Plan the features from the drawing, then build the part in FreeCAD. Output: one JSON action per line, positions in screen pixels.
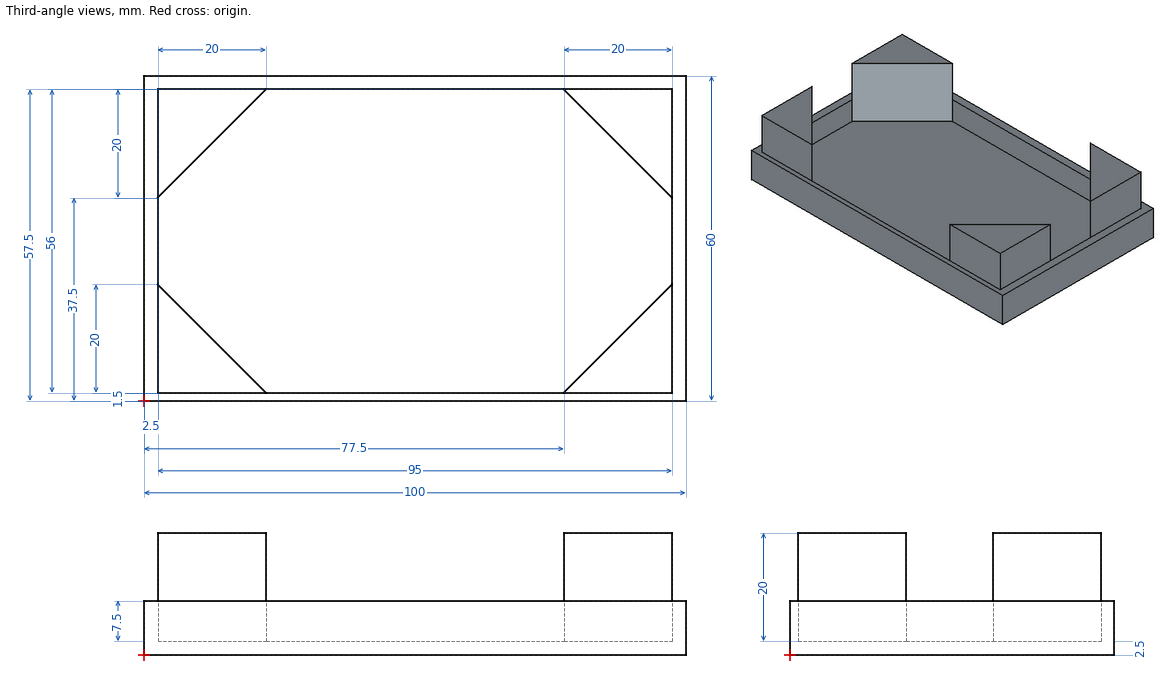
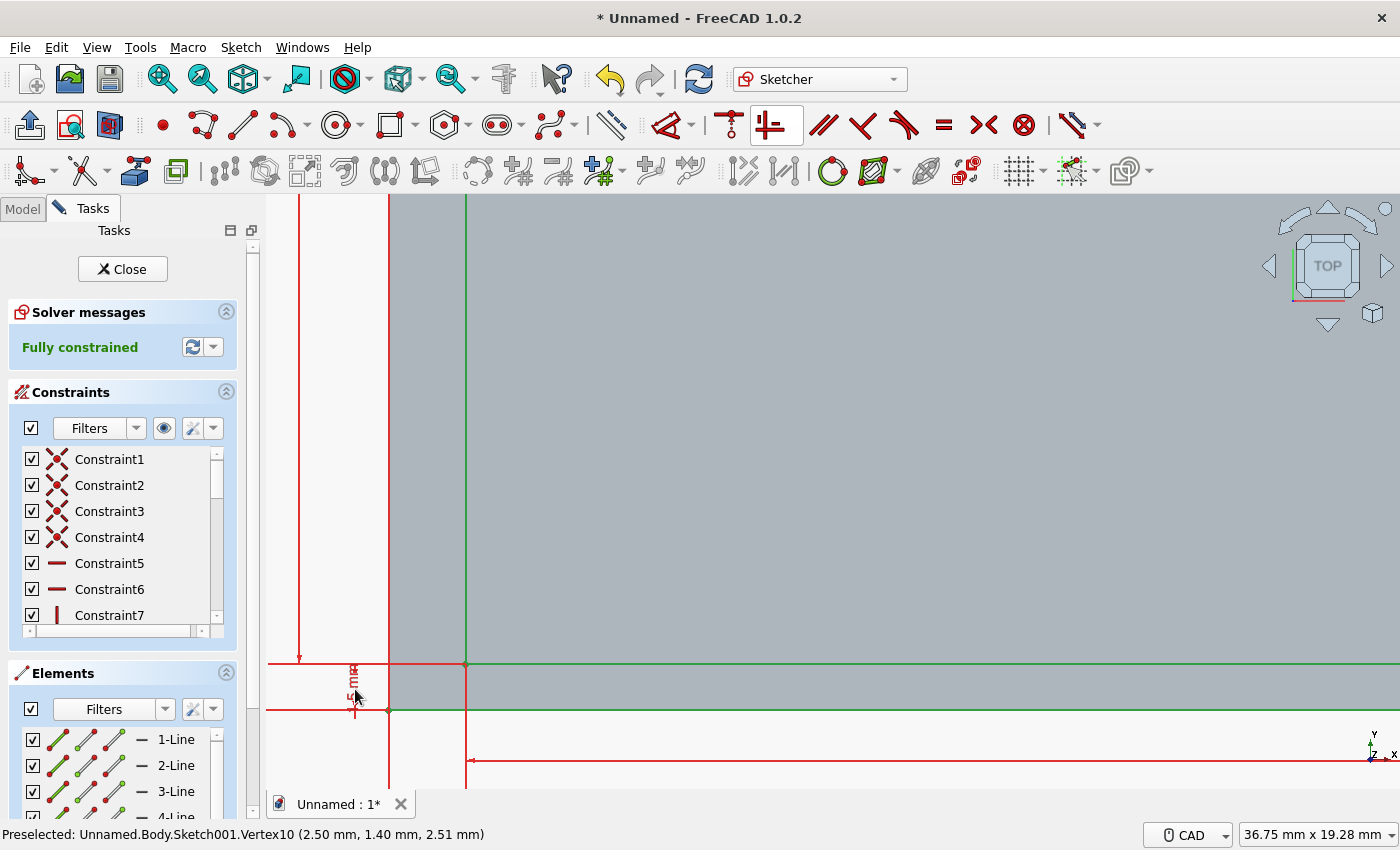
{"action": "left_click", "coordinate": [123, 269]}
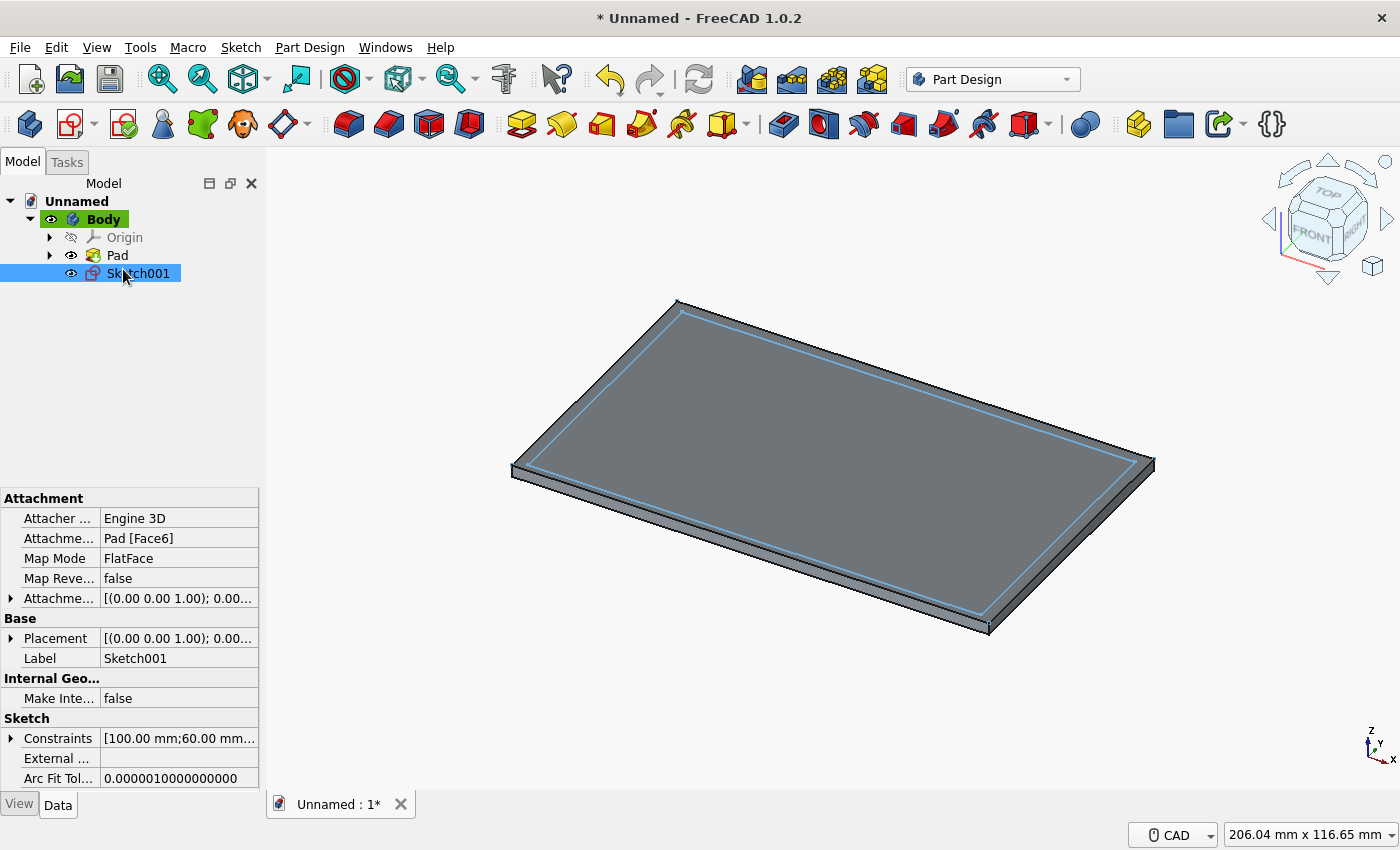
{"action": "left_click", "coordinate": [522, 124]}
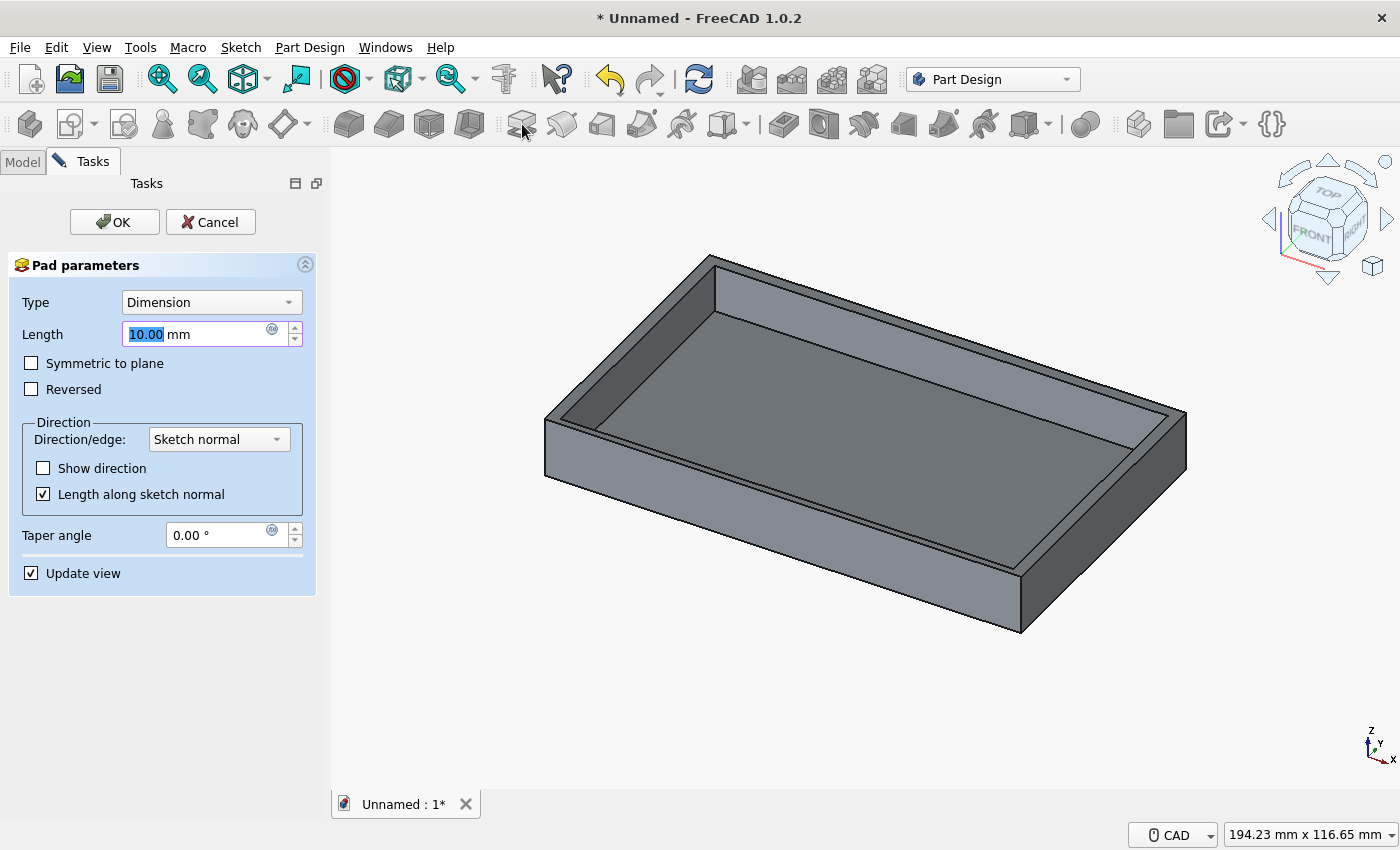
{"action": "type", "text": "7.5"}
{"action": "key", "text": "Tab"}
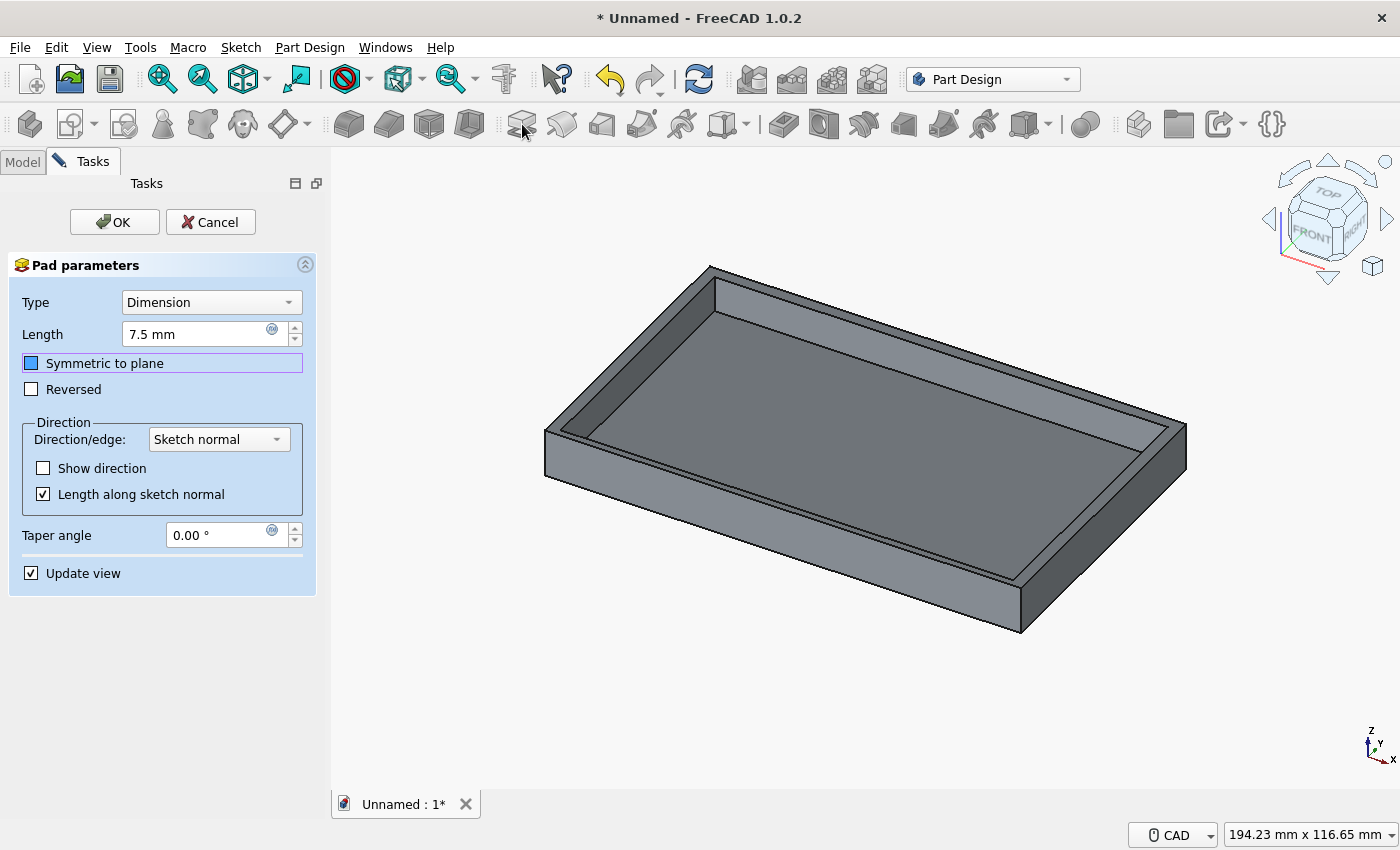
{"action": "left_click", "coordinate": [115, 222]}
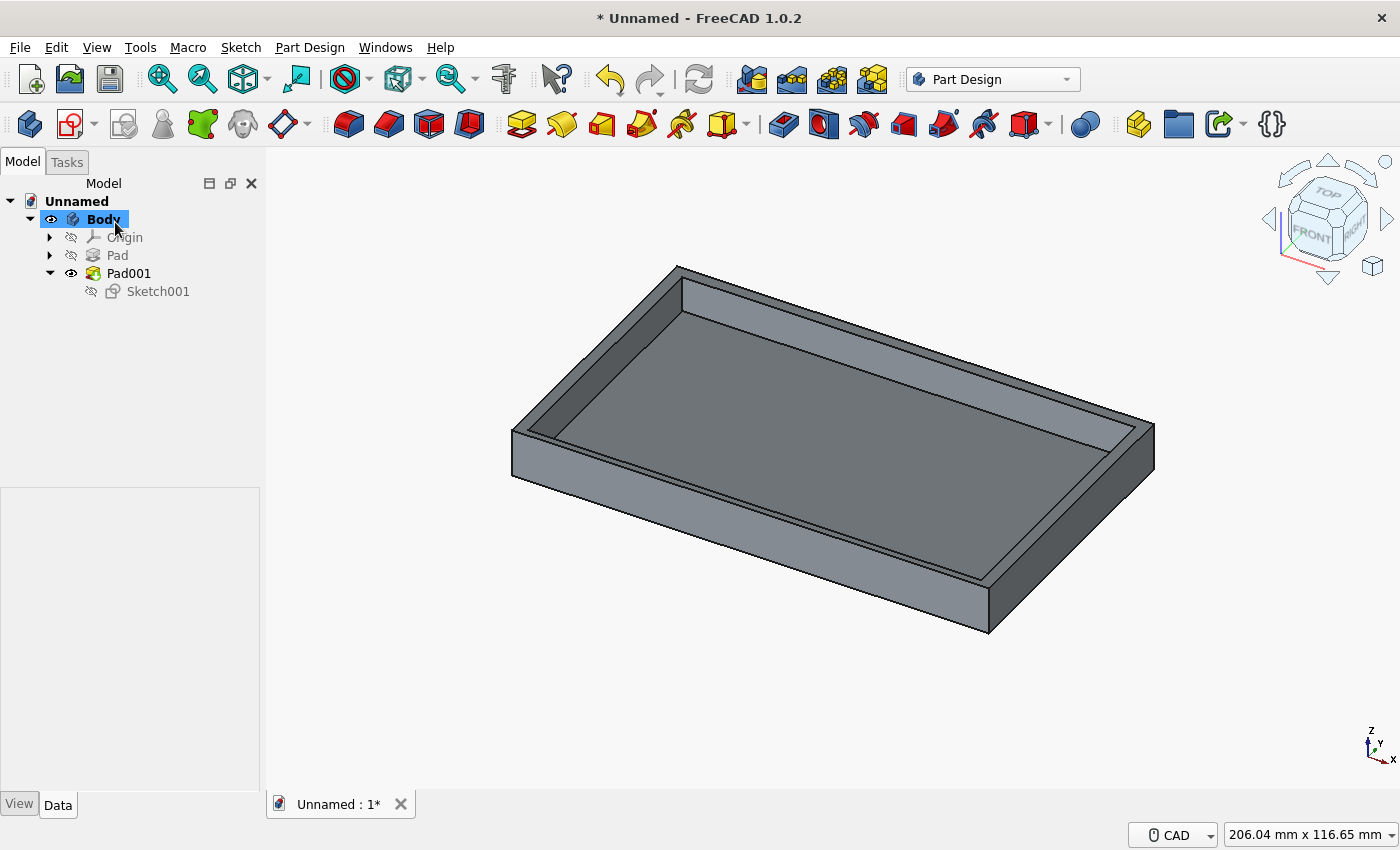
{"action": "left_click", "coordinate": [896, 483]}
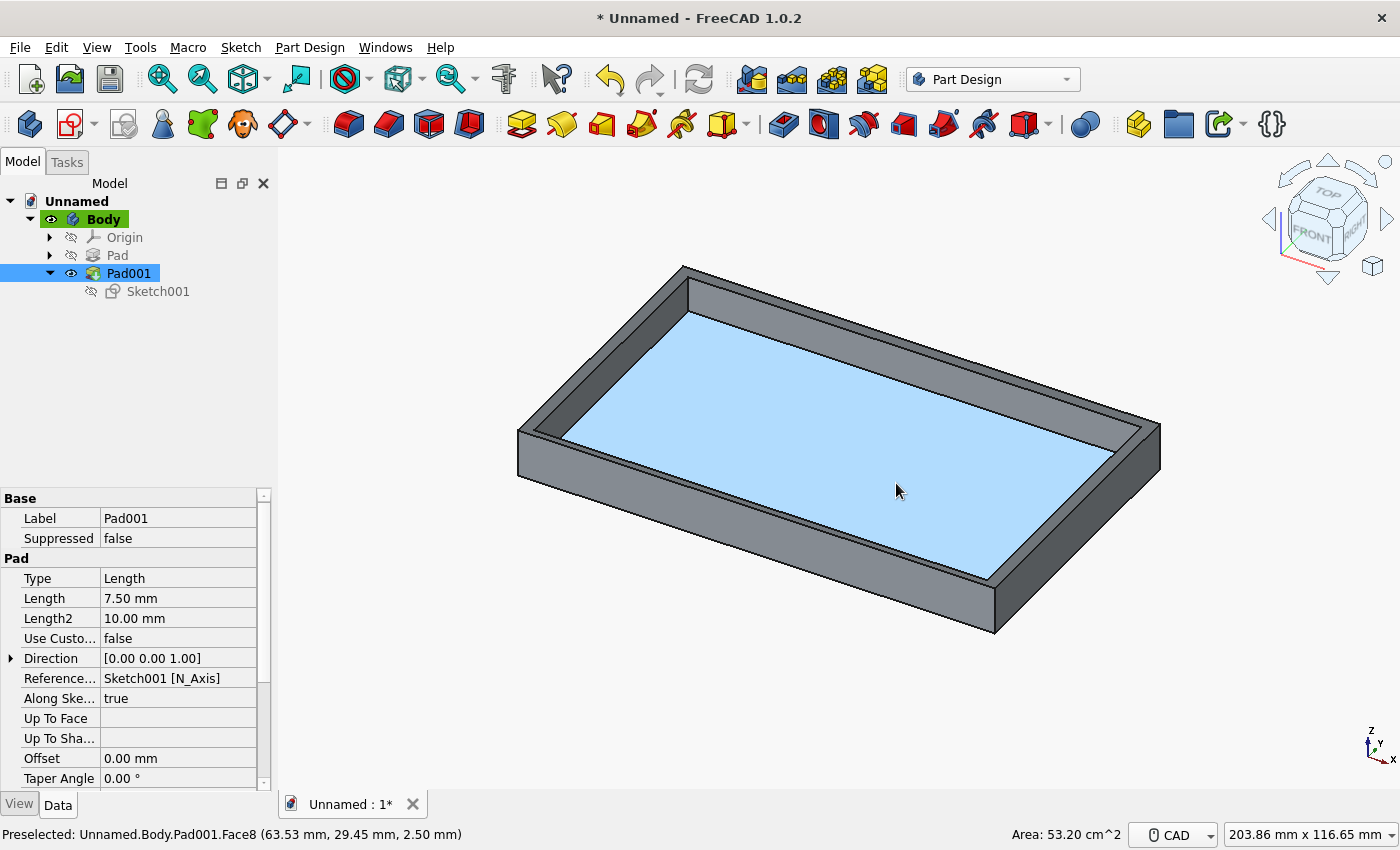
{"action": "left_click", "coordinate": [70, 124]}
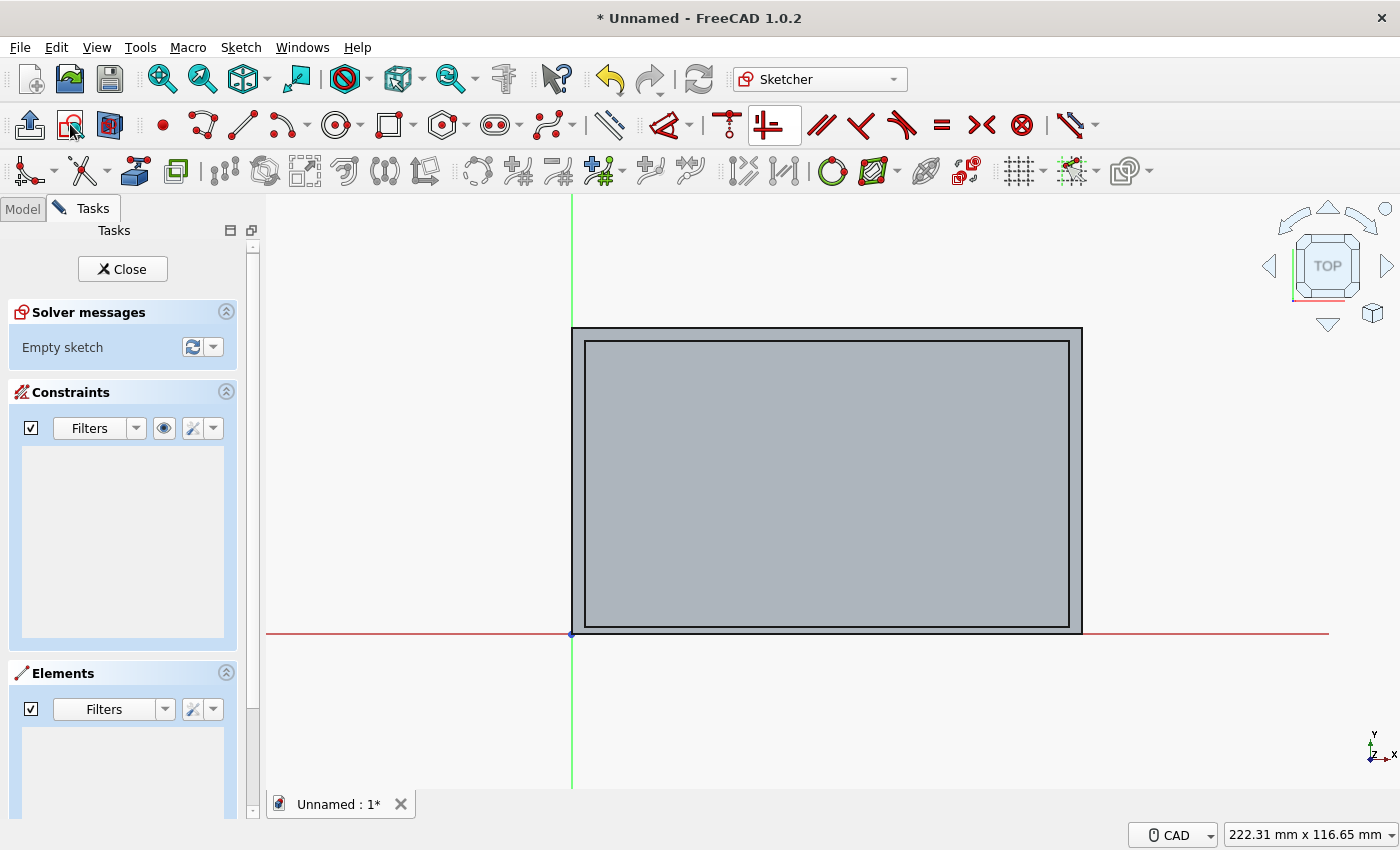
{"action": "left_click", "coordinate": [204, 126]}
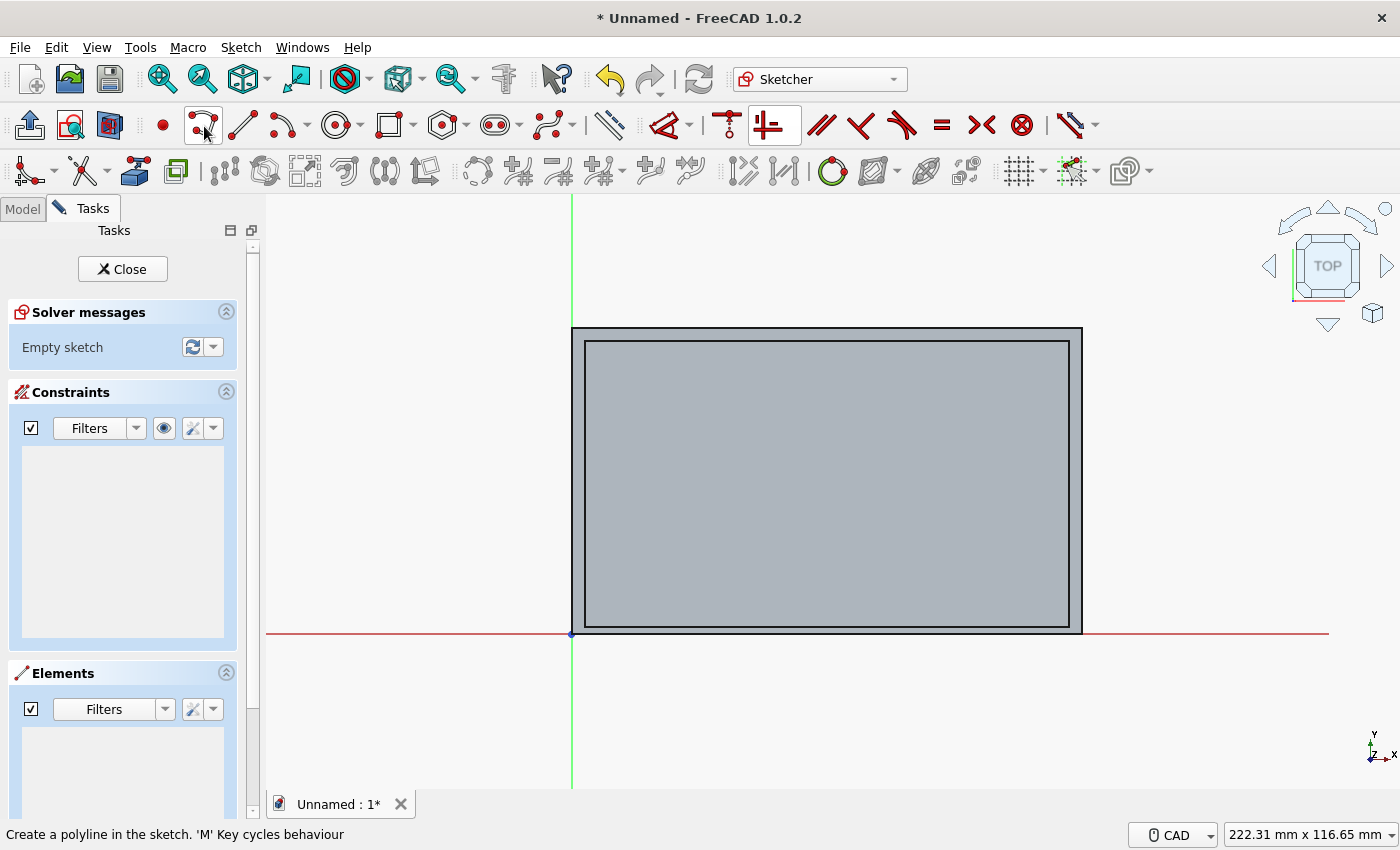
{"action": "scroll", "coordinate": [585, 443], "scroll_direction": "up", "scroll_amount": 2}